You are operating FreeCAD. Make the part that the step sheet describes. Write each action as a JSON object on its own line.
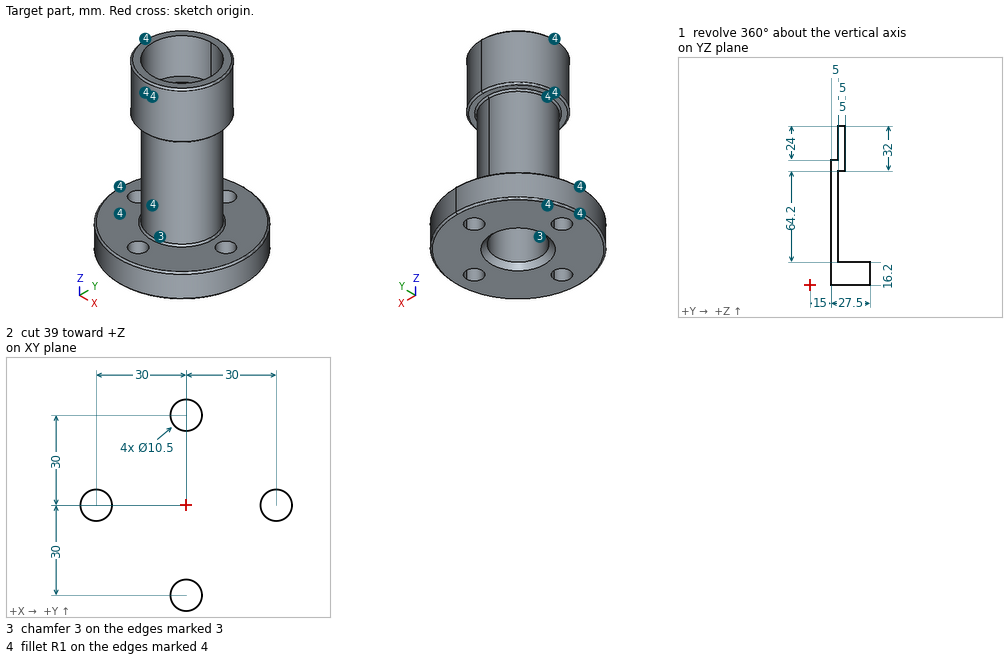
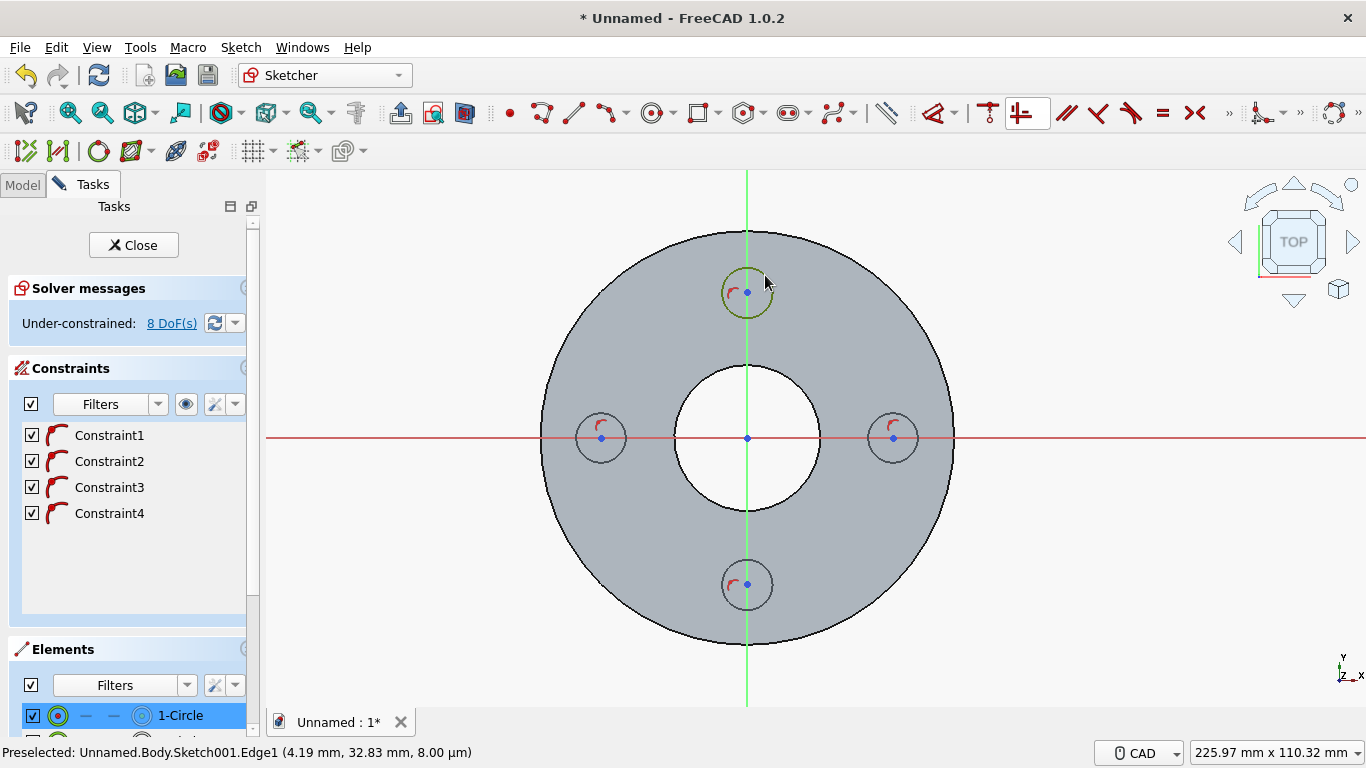
{"action": "left_click", "coordinate": [618, 420]}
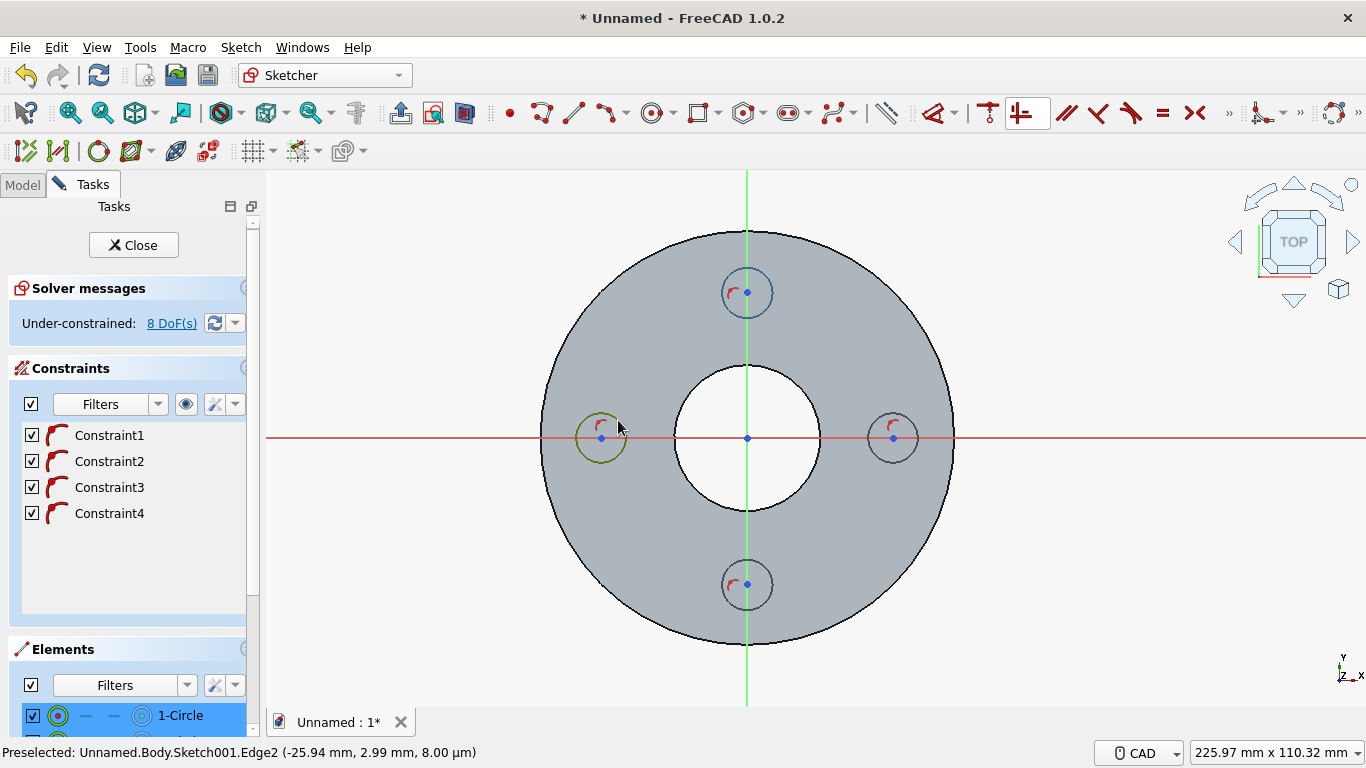
{"action": "left_click", "coordinate": [765, 567]}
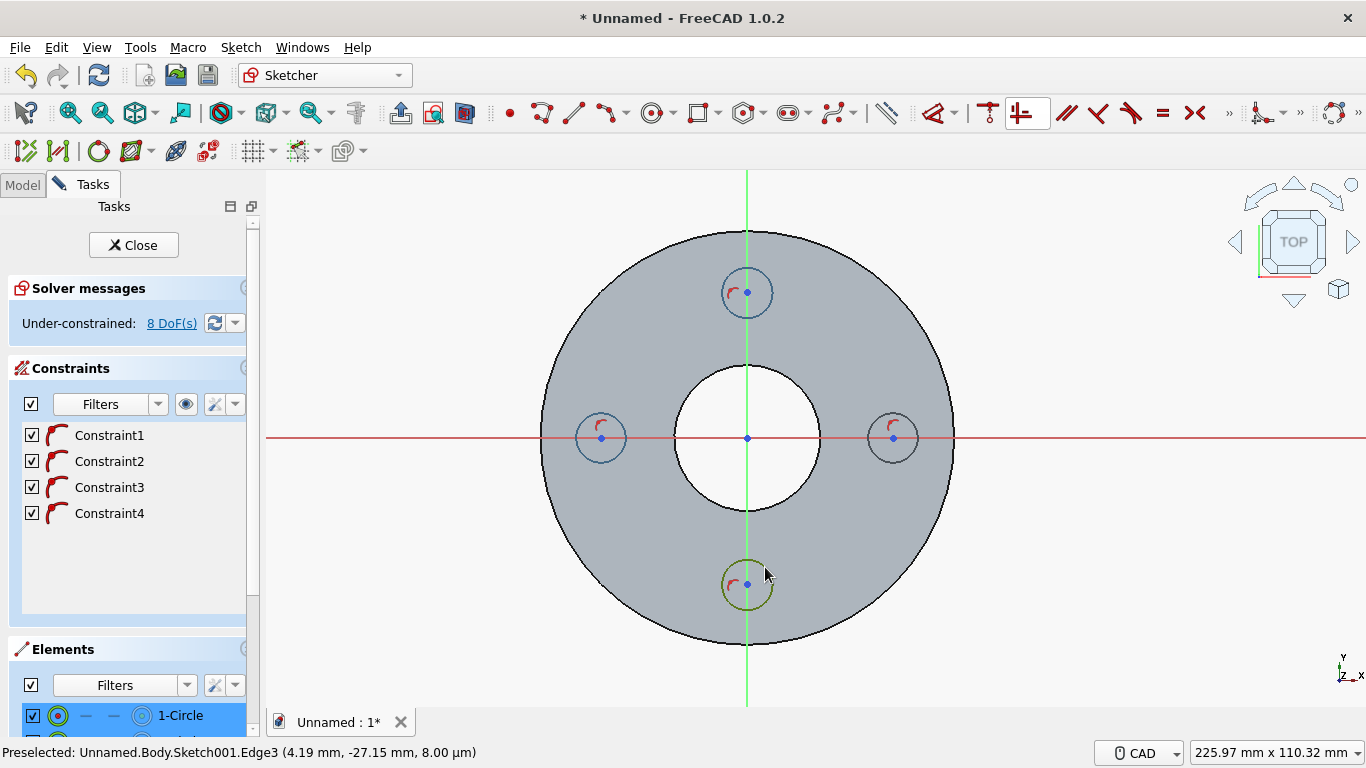
{"action": "left_click", "coordinate": [910, 420]}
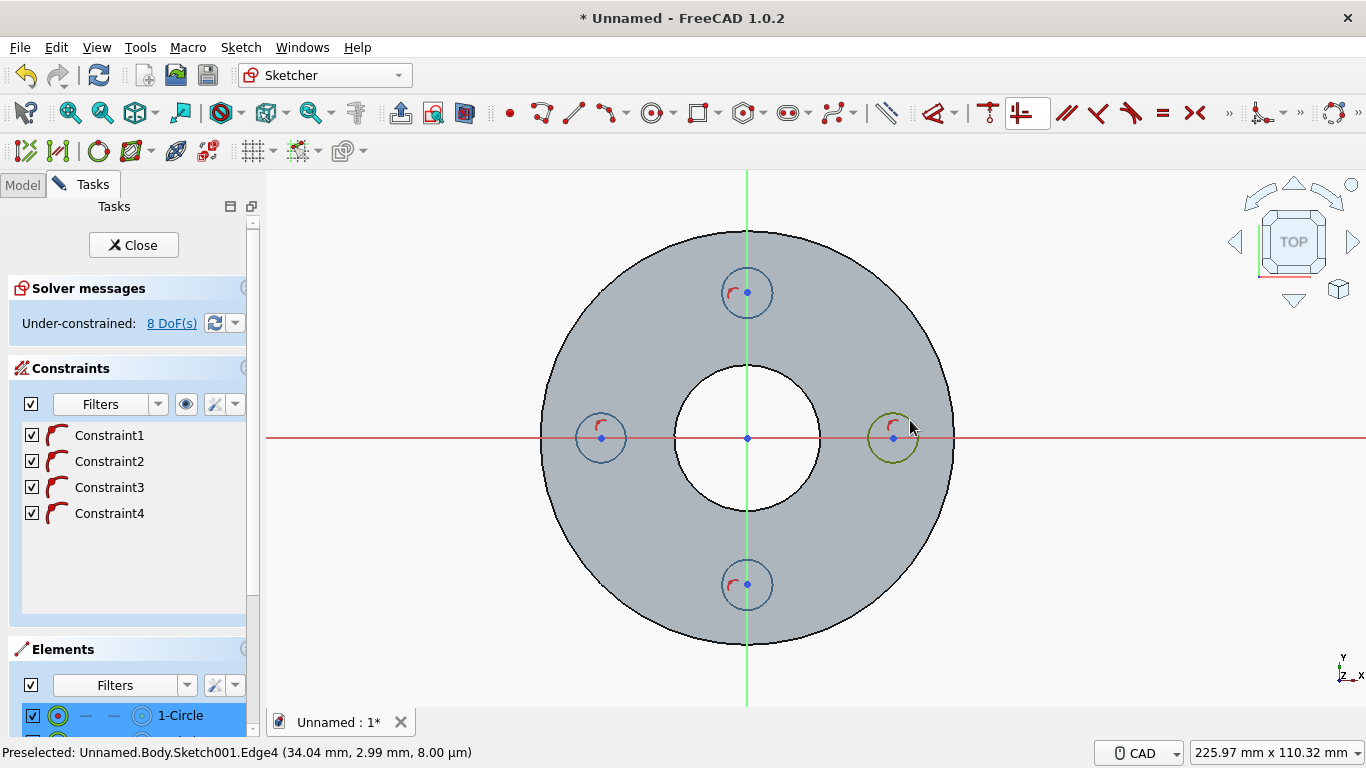
{"action": "left_click", "coordinate": [1164, 114]}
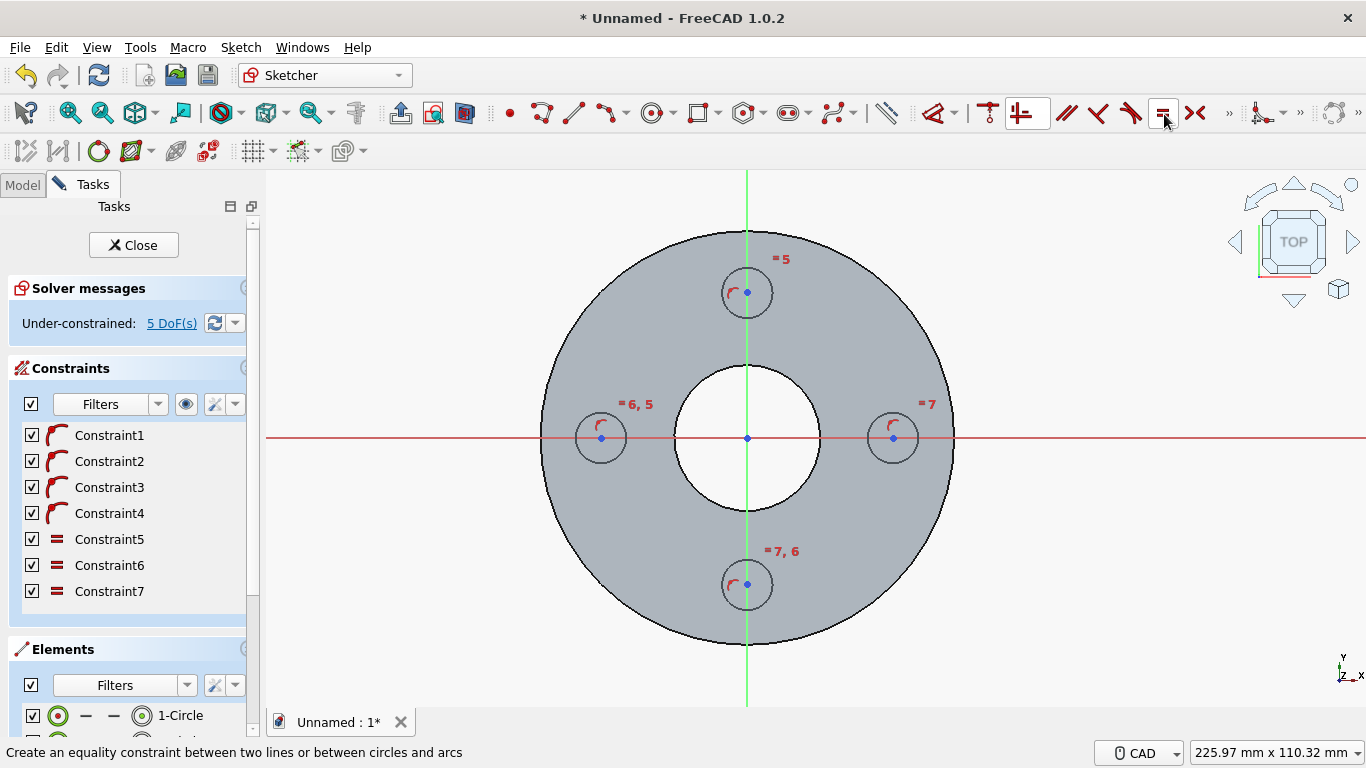
{"action": "left_click", "coordinate": [934, 114]}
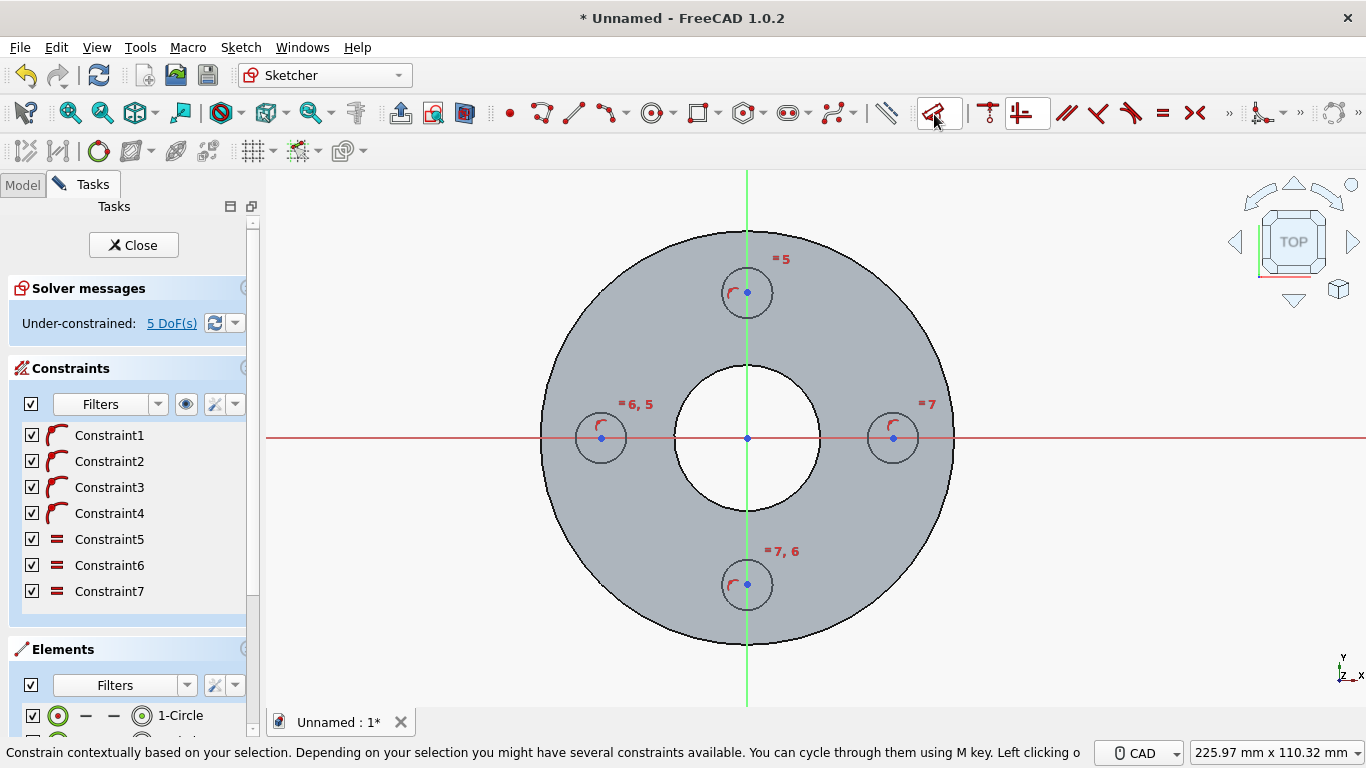
{"action": "left_click", "coordinate": [765, 275]}
{"action": "left_click", "coordinate": [787, 252]}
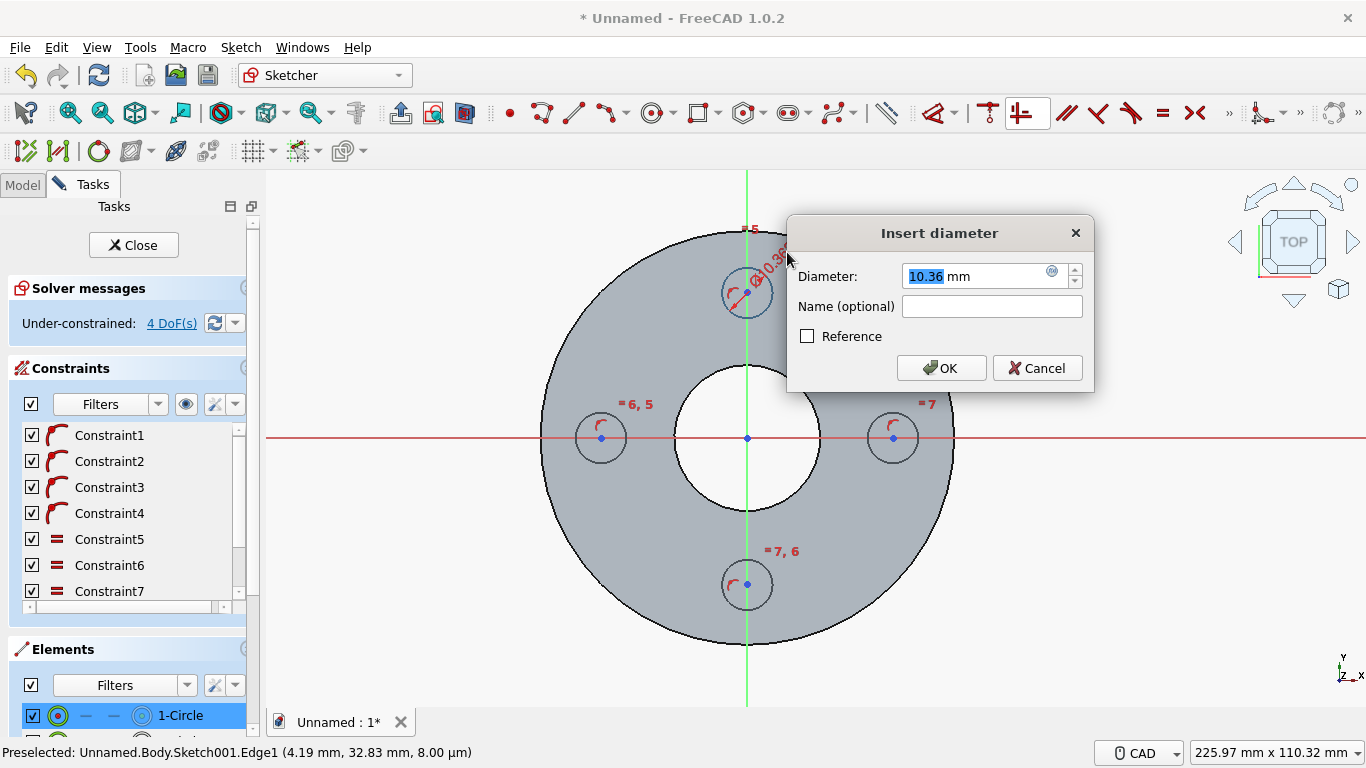
{"action": "type", "text": "10.5"}
{"action": "key", "text": "Return"}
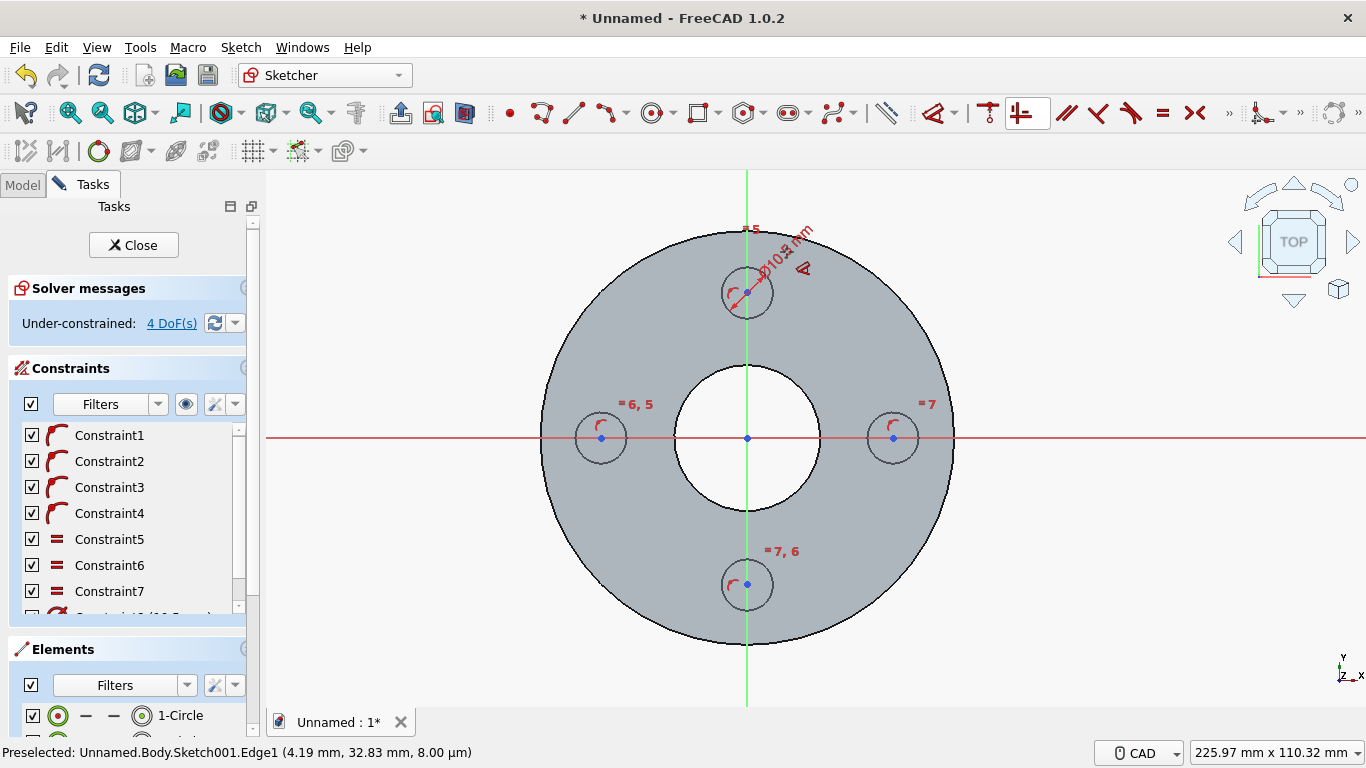
{"action": "left_click", "coordinate": [747, 293]}
{"action": "left_click", "coordinate": [781, 366]}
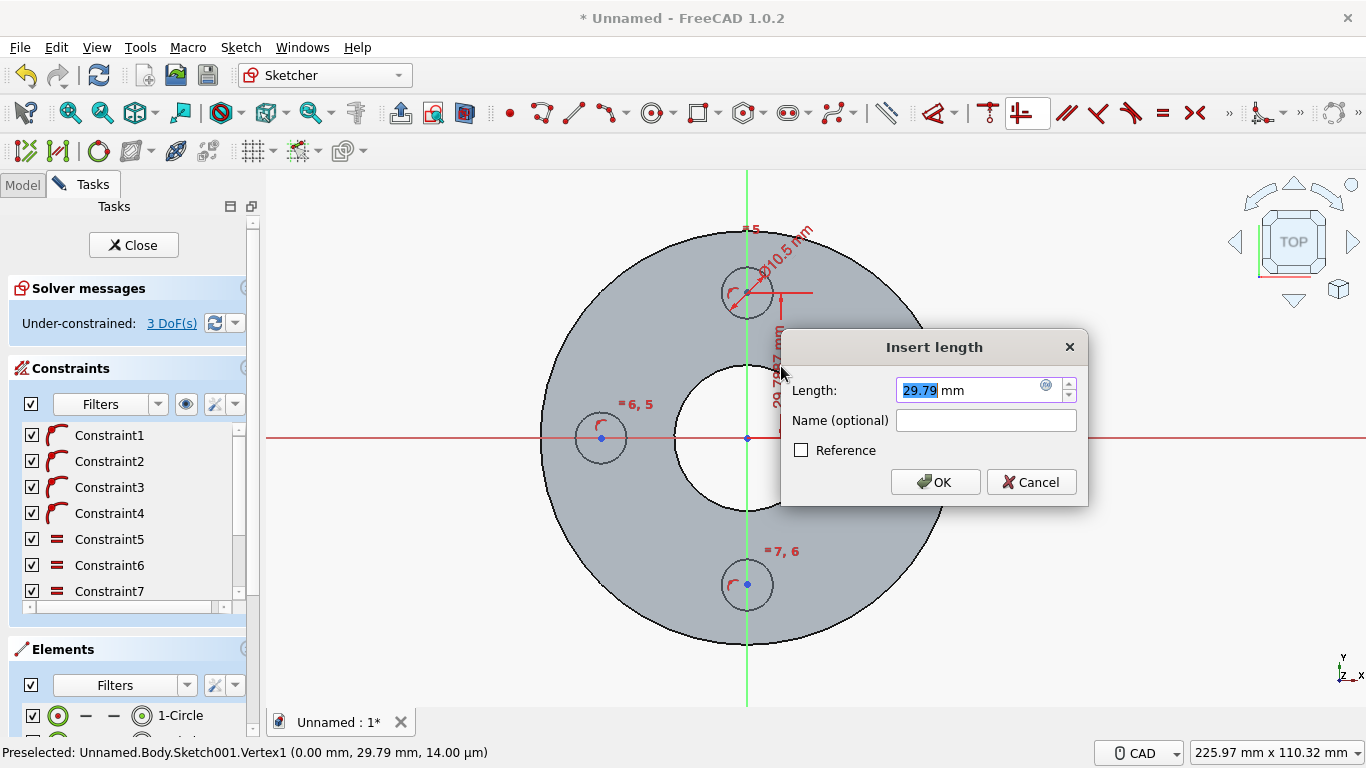
{"action": "type", "text": "30"}
{"action": "key", "text": "Return"}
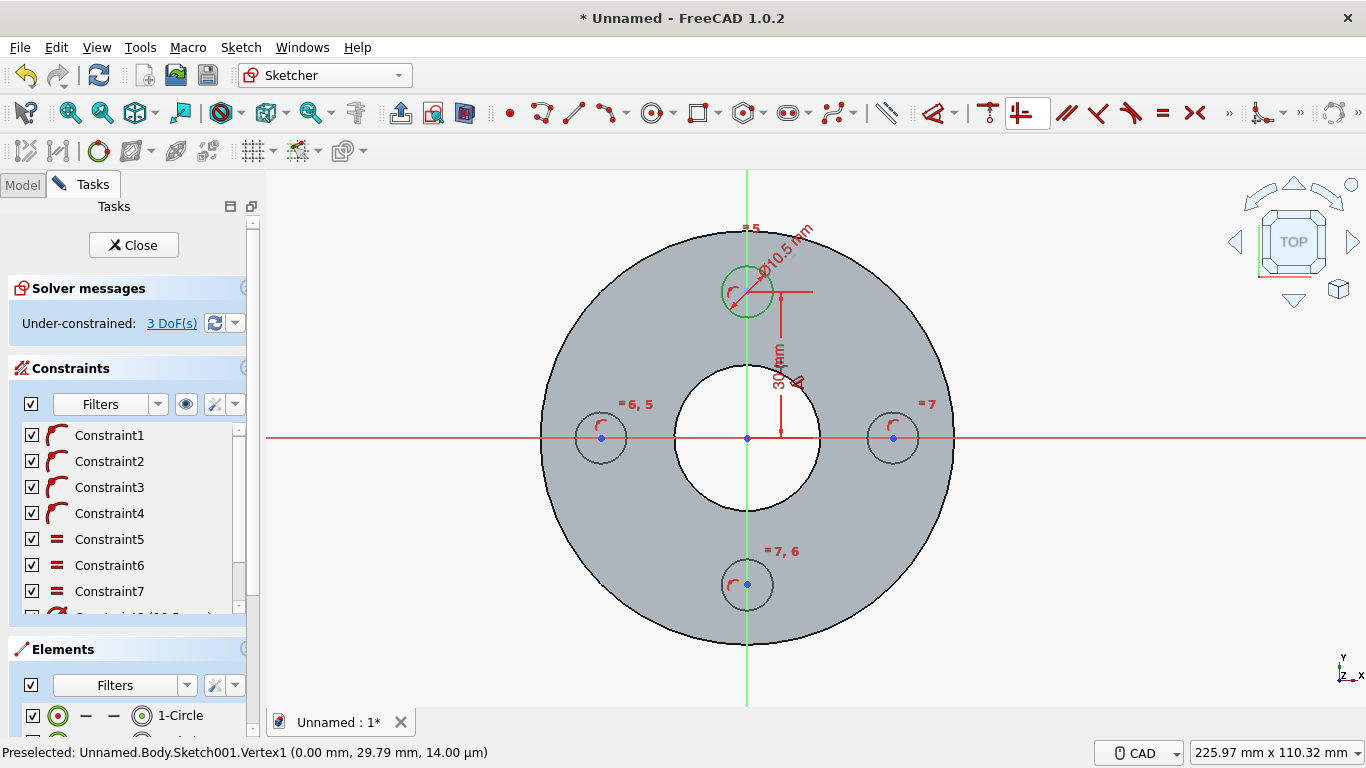
{"action": "left_click", "coordinate": [601, 438]}
{"action": "left_click", "coordinate": [674, 472]}